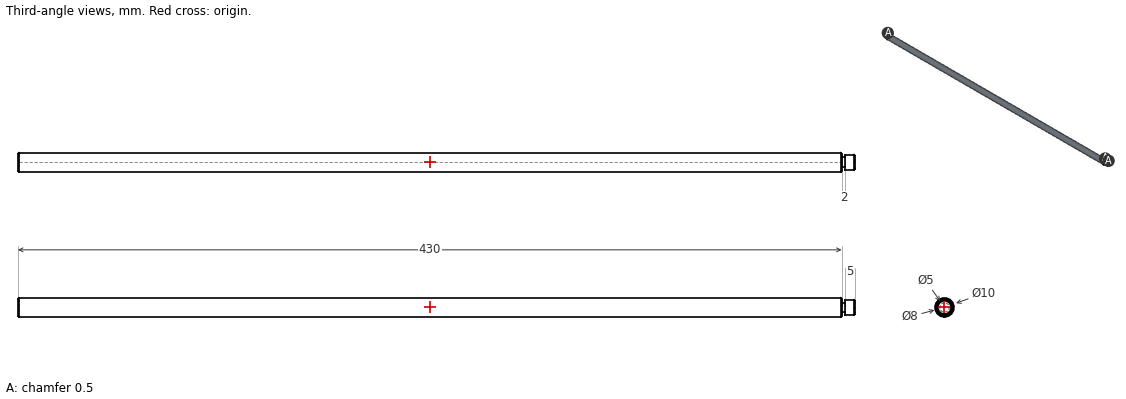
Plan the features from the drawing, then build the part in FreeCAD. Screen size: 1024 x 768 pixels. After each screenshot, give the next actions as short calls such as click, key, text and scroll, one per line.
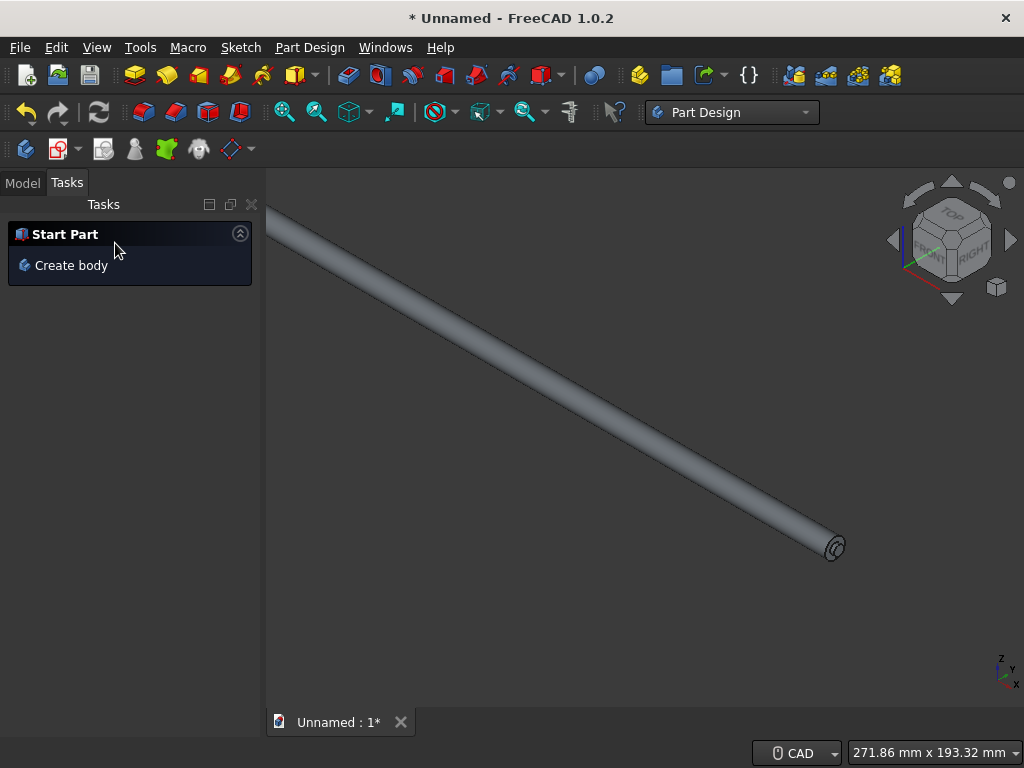
click(286, 112)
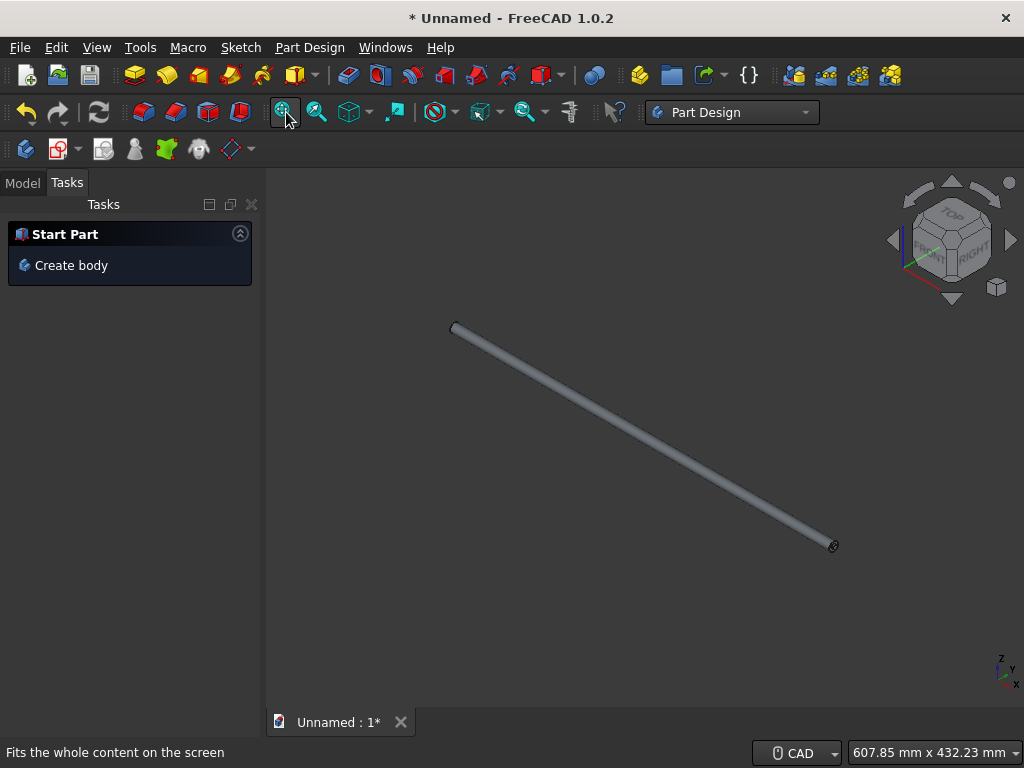
scroll(835, 546, up, 7)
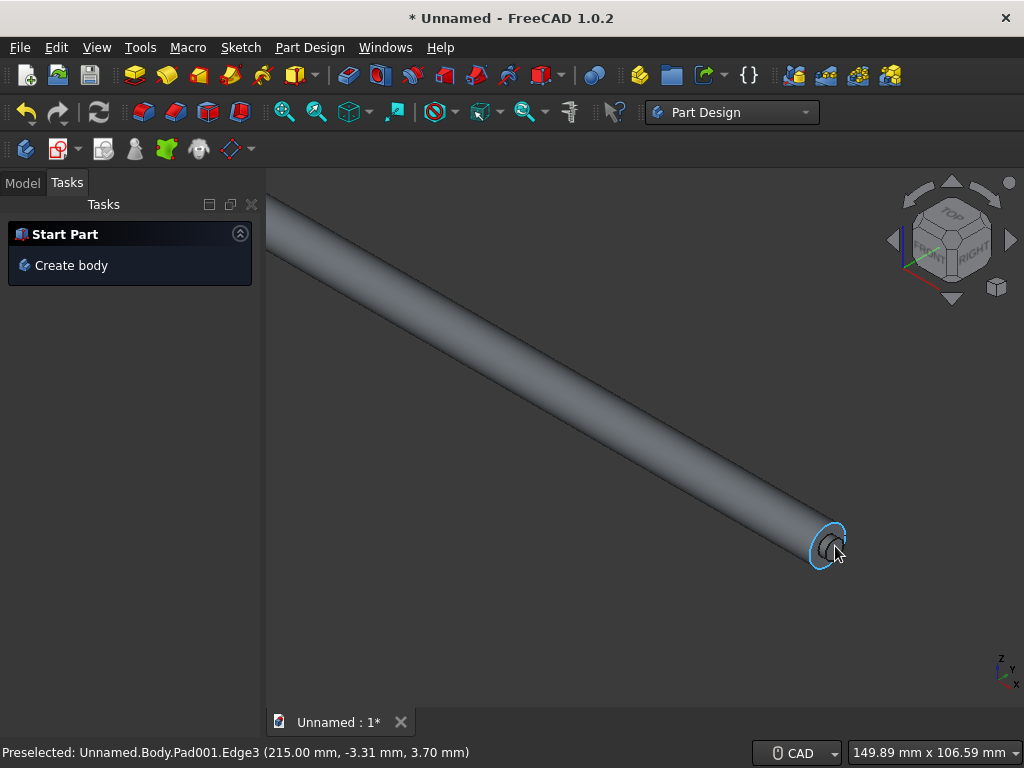
click(286, 112)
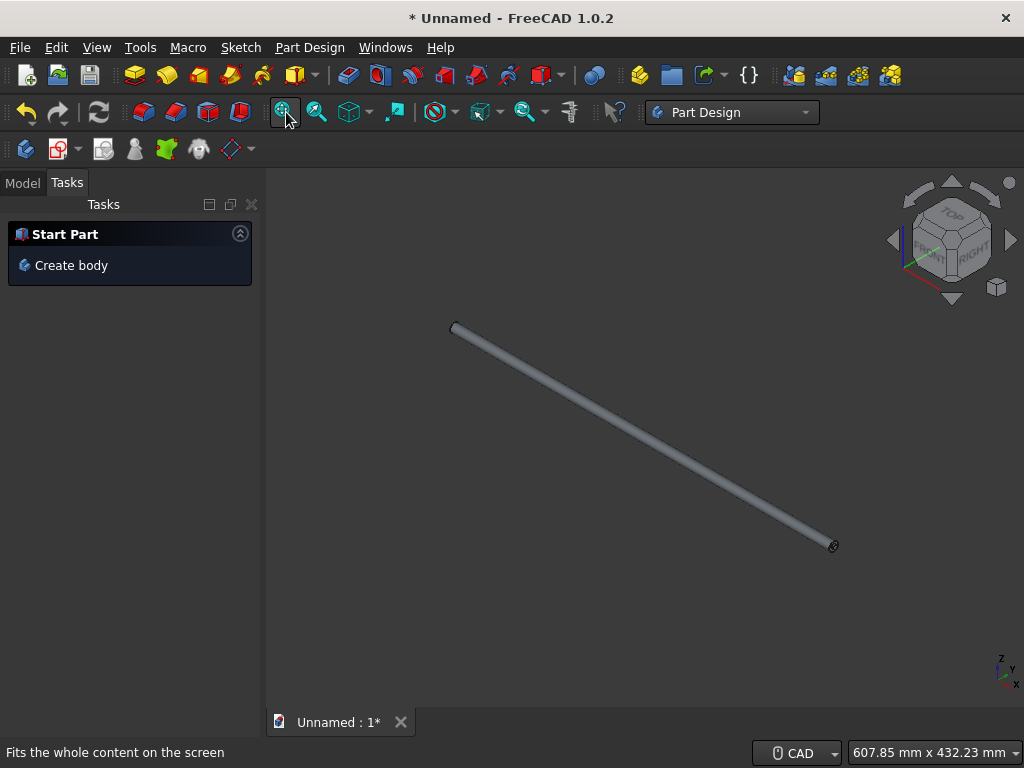
key(3)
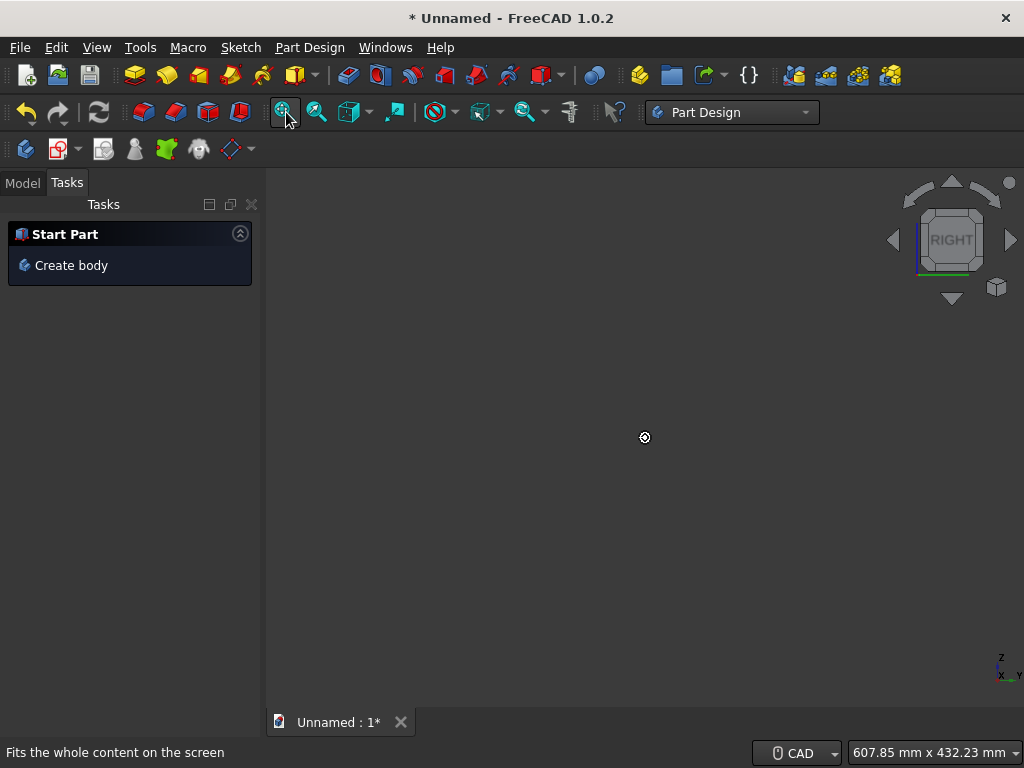
key(v)
key(f)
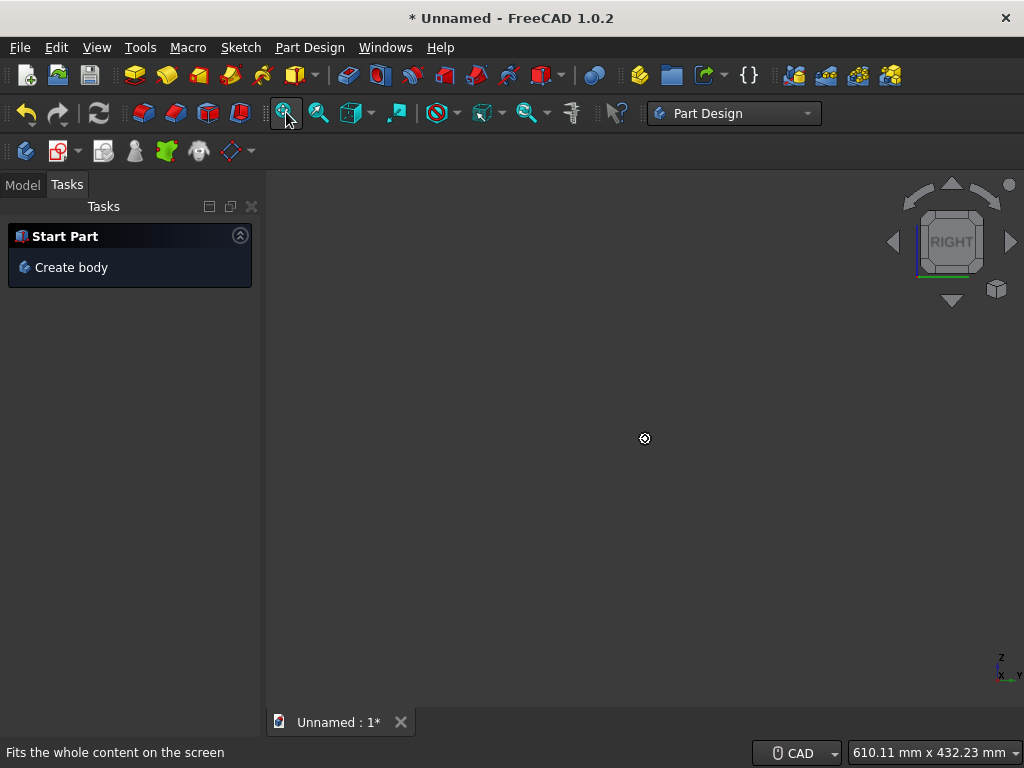
scroll(645, 437, up, 7)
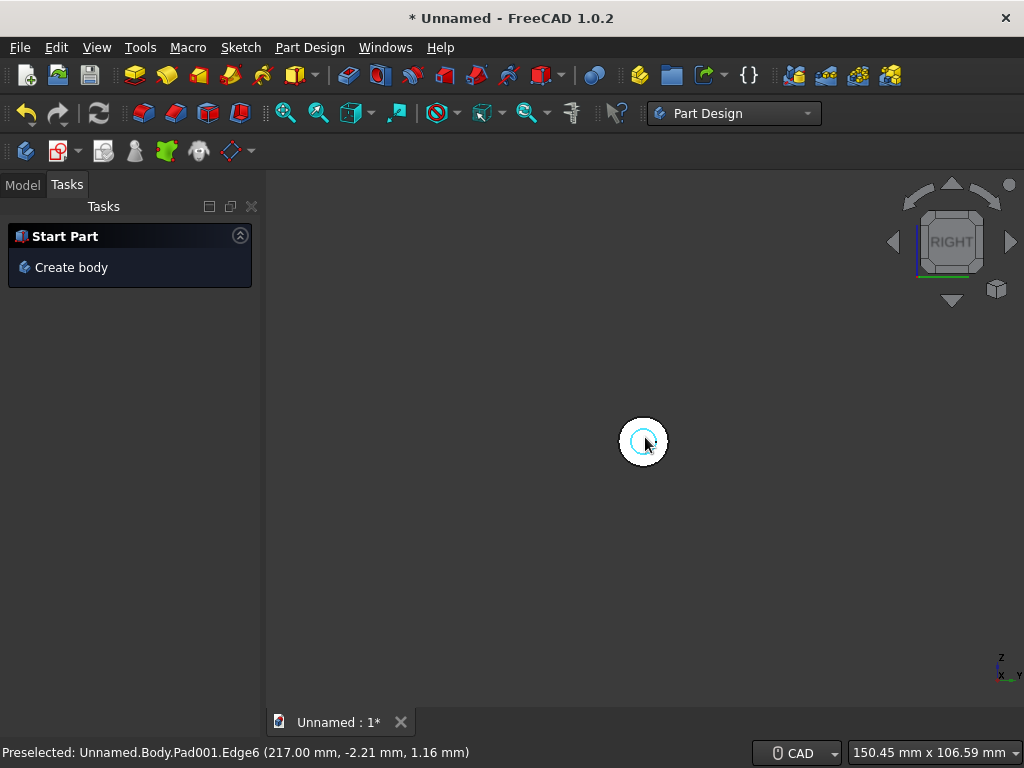
click(643, 441)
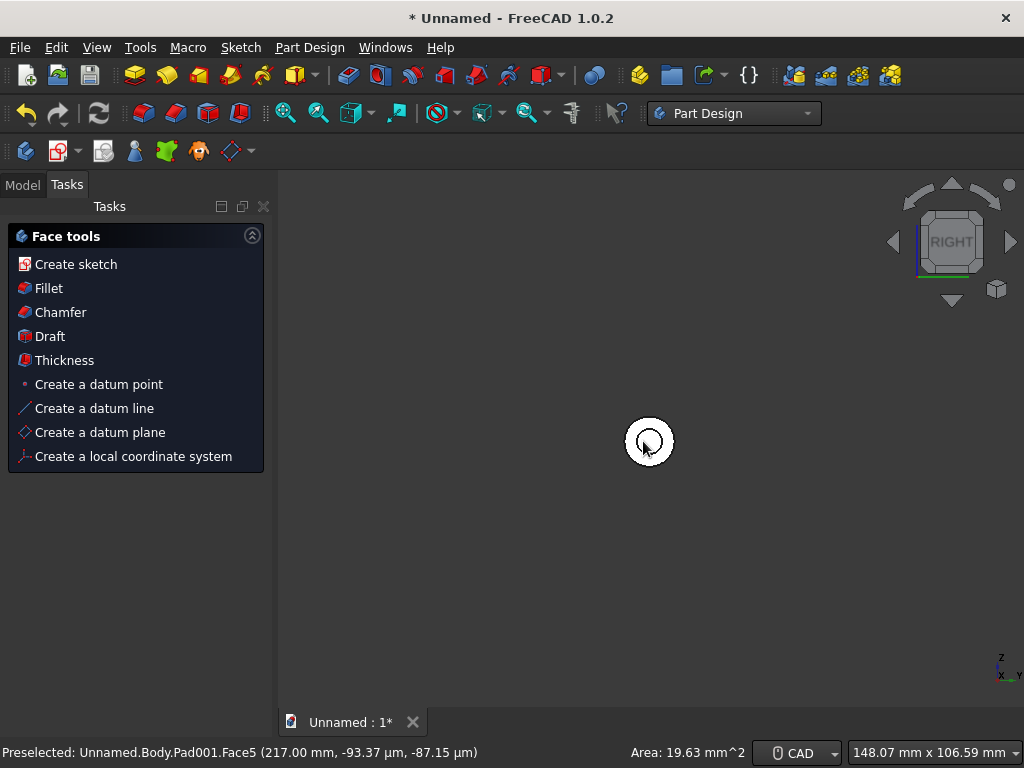
click(58, 152)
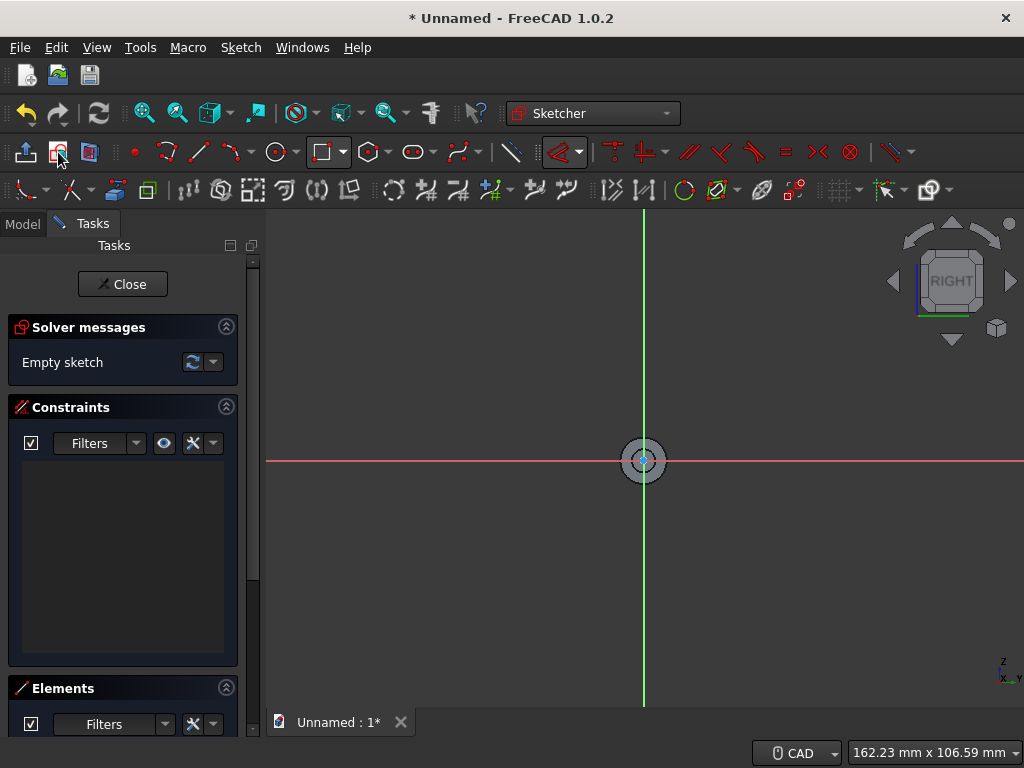
scroll(652, 461, up, 11)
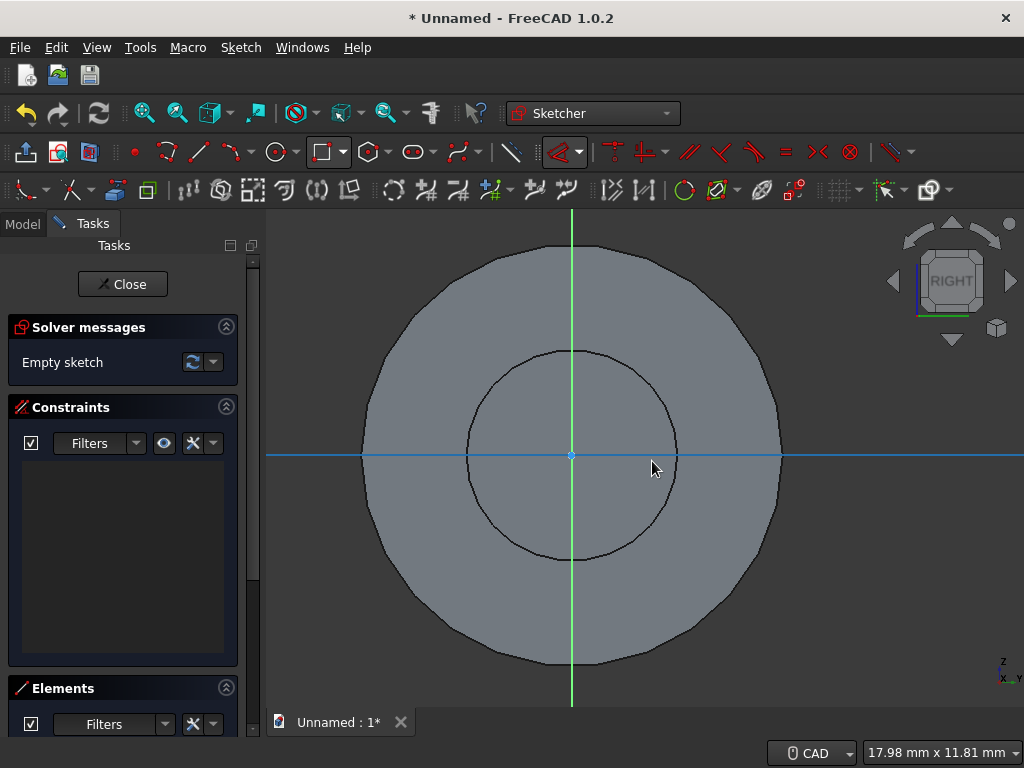
click(276, 152)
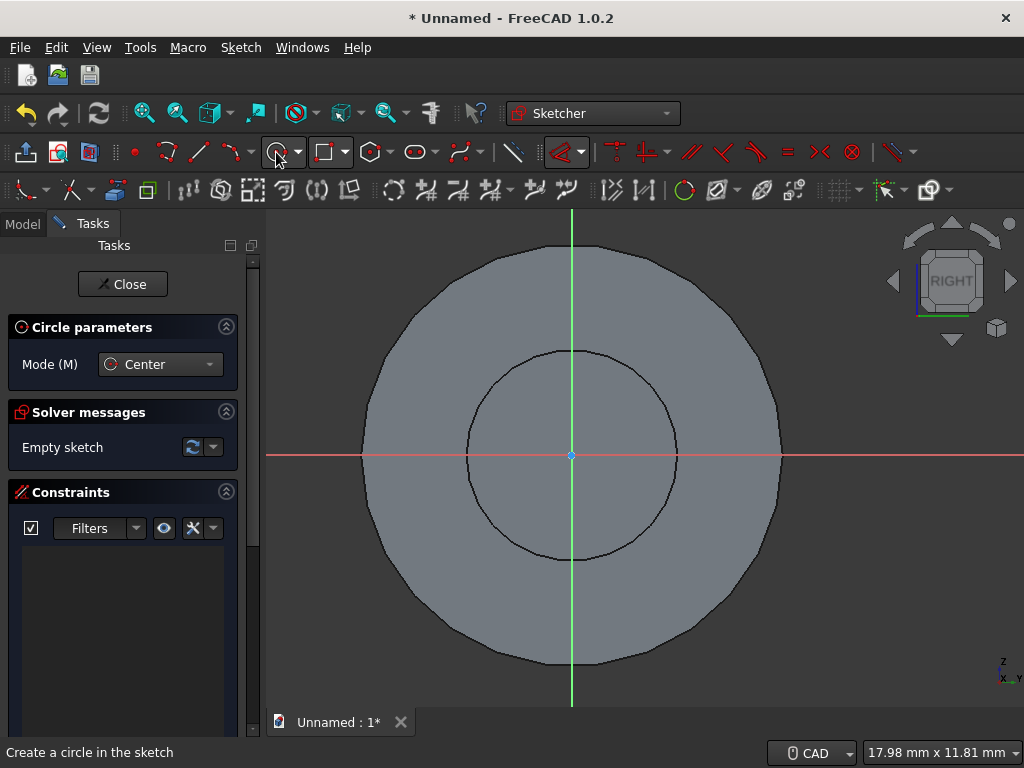
click(572, 455)
move(691, 336)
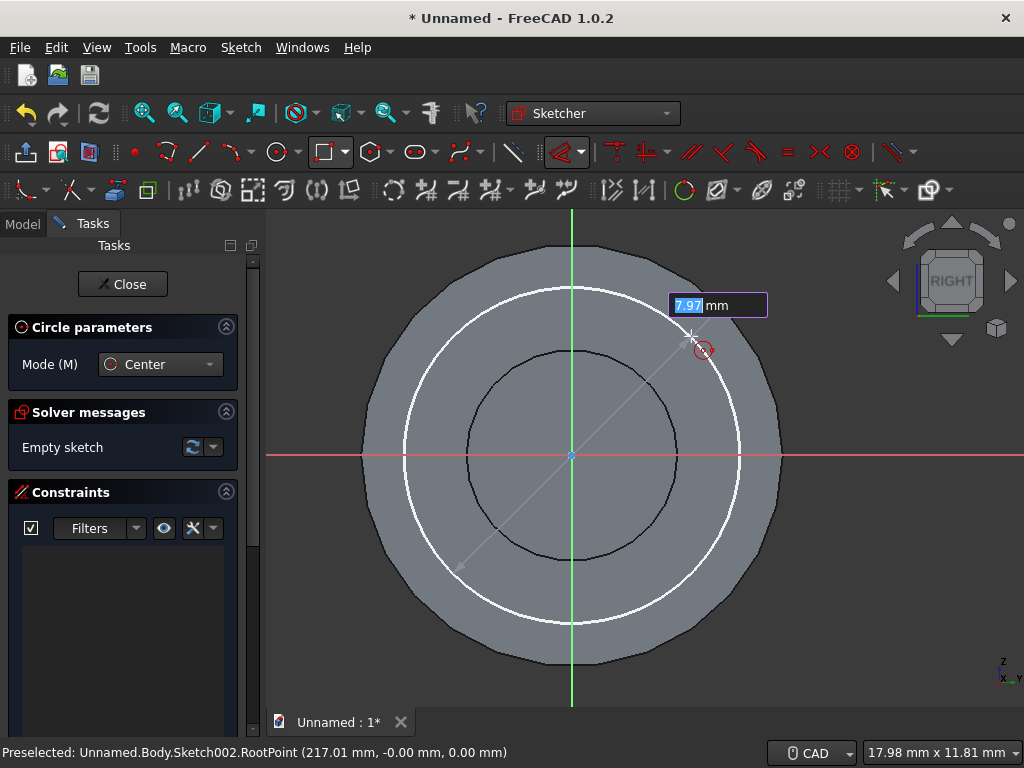
text(8)
key(Return)
key(Escape)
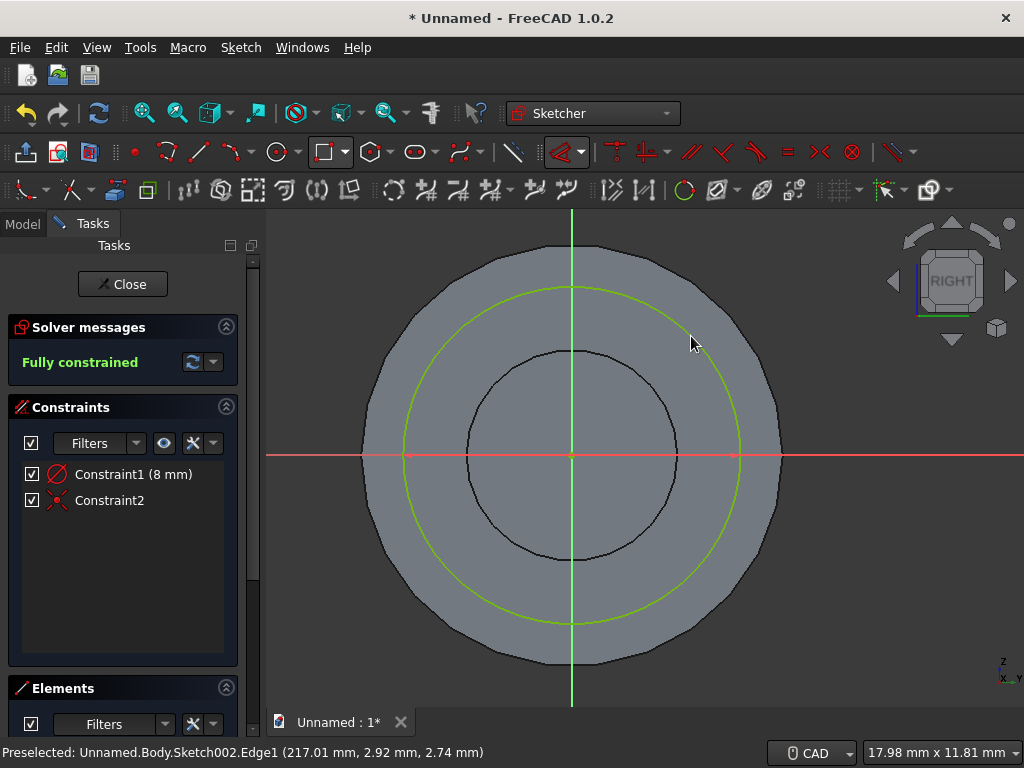
click(123, 284)